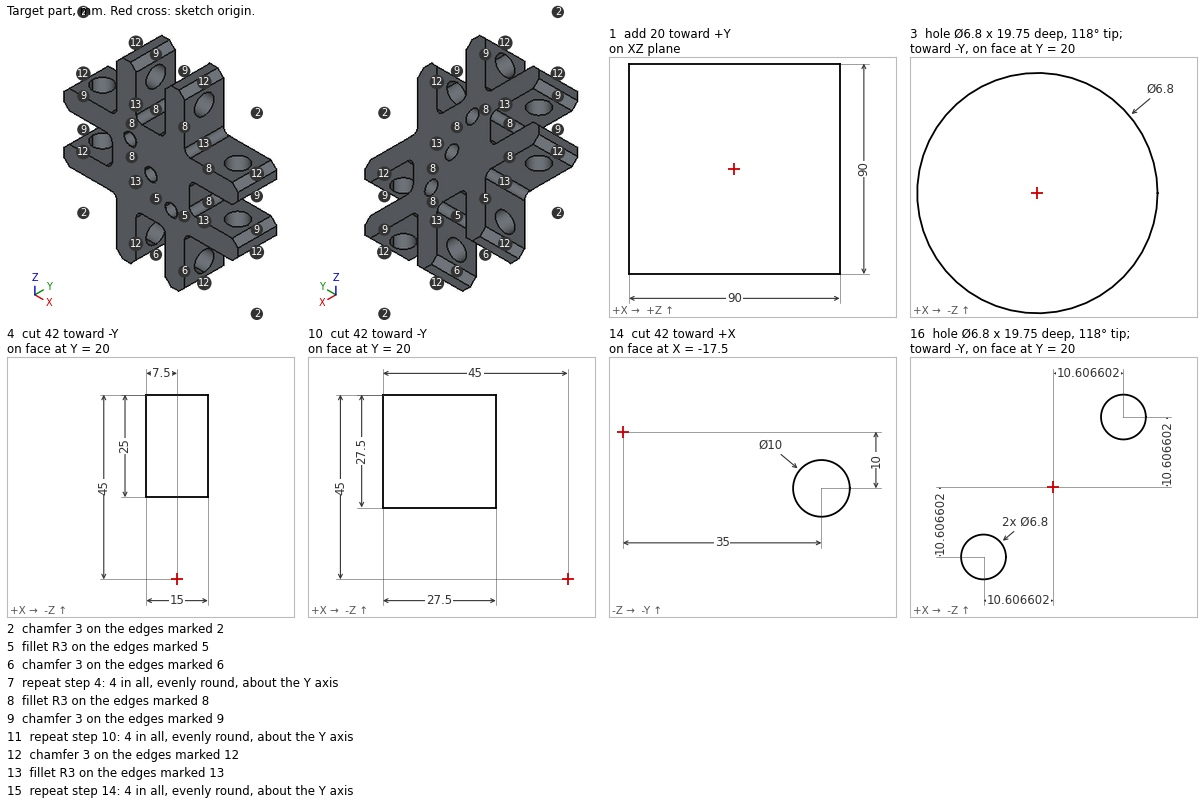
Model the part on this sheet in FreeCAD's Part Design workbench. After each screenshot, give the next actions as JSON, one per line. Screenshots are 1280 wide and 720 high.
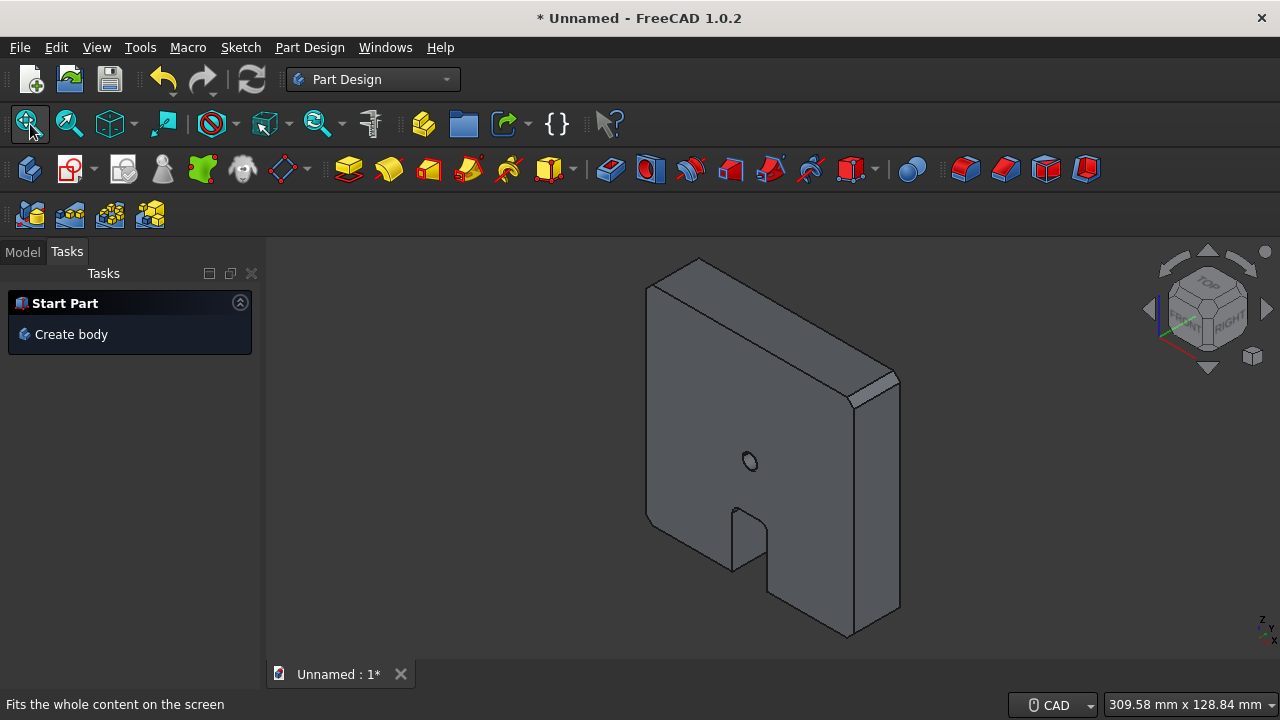
{"action": "key", "text": "1"}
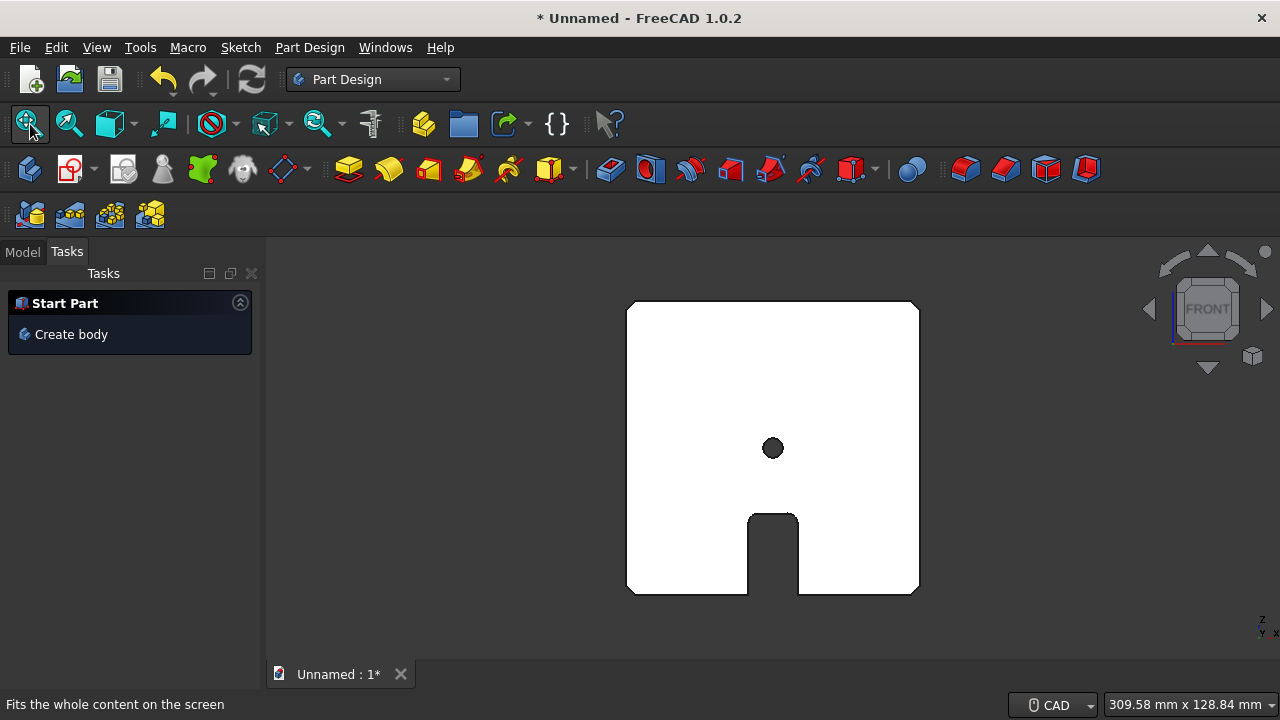
{"action": "key", "text": "3"}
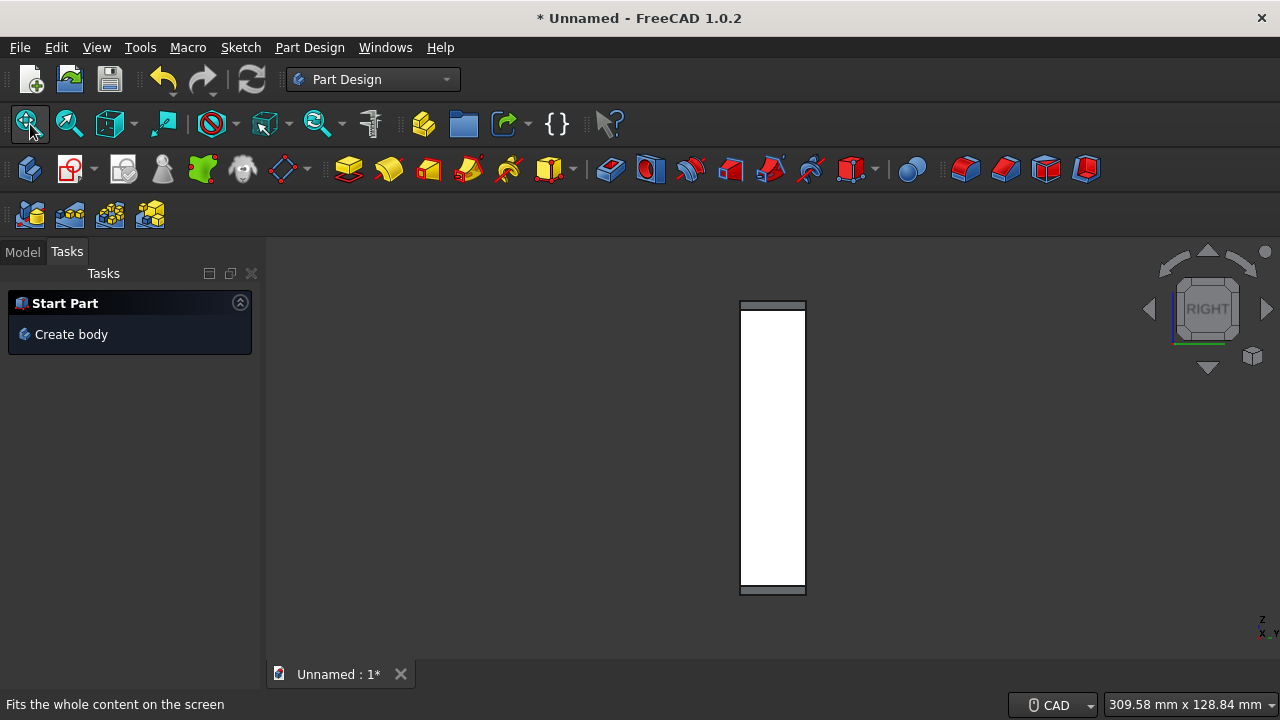
{"action": "key", "text": "5"}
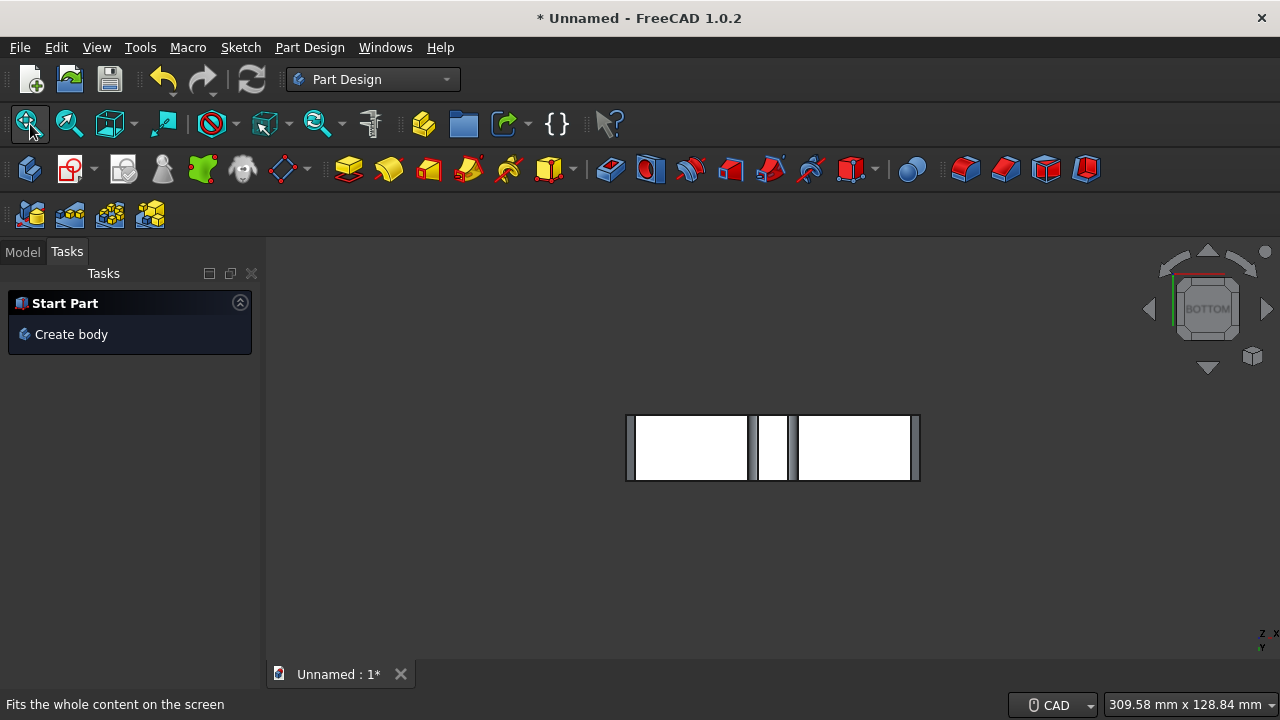
{"action": "left_click", "coordinate": [30, 124]}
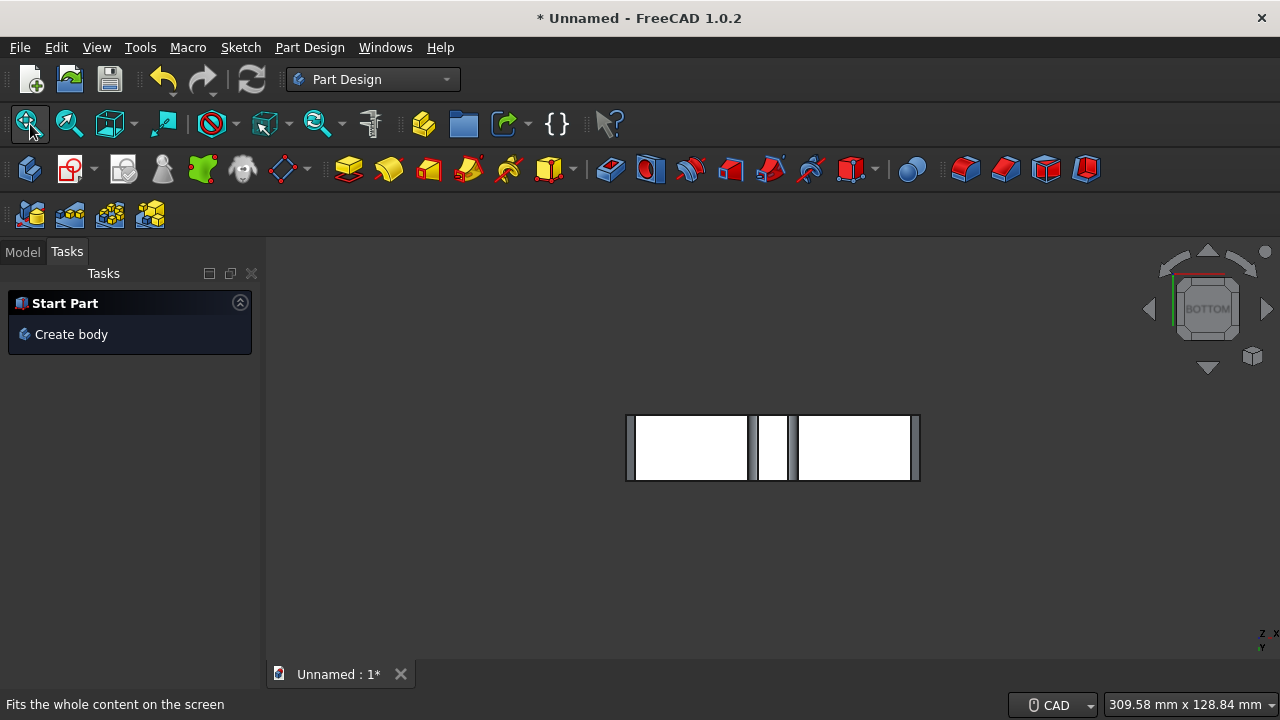
{"action": "left_click", "coordinate": [798, 447]}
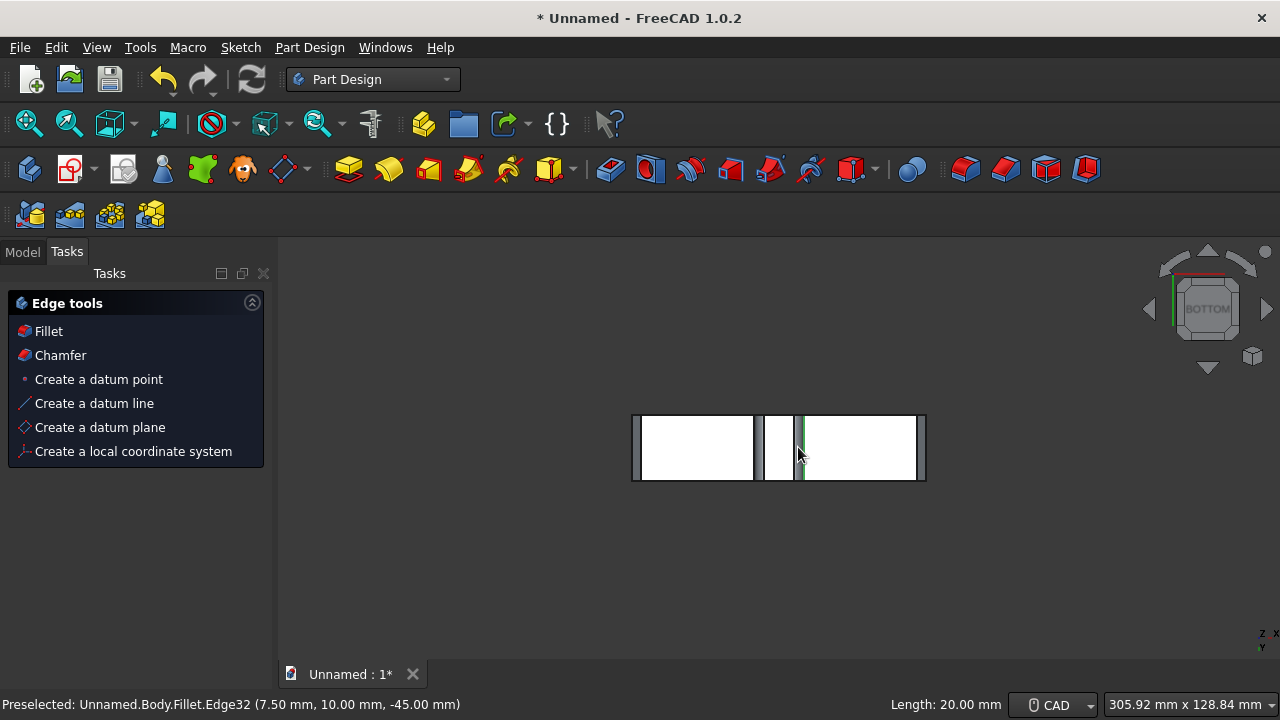
{"action": "left_click", "coordinate": [754, 447], "text": "ctrl"}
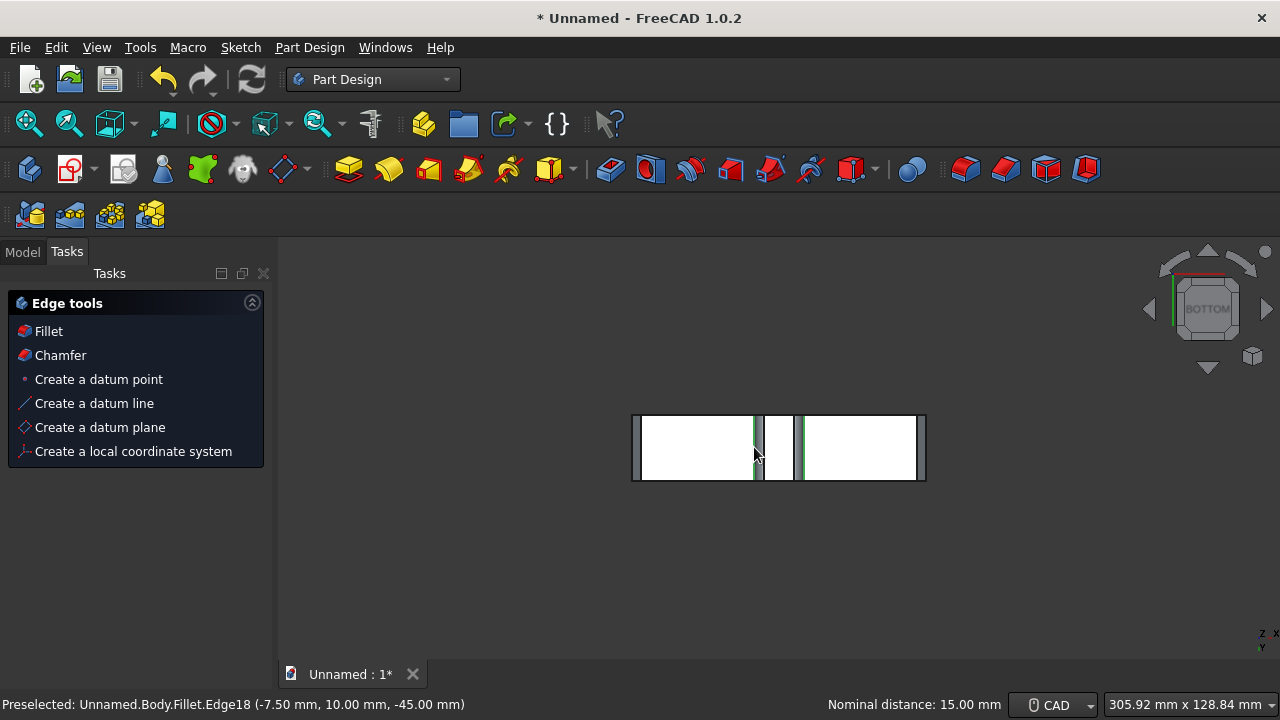
{"action": "left_click", "coordinate": [1006, 170]}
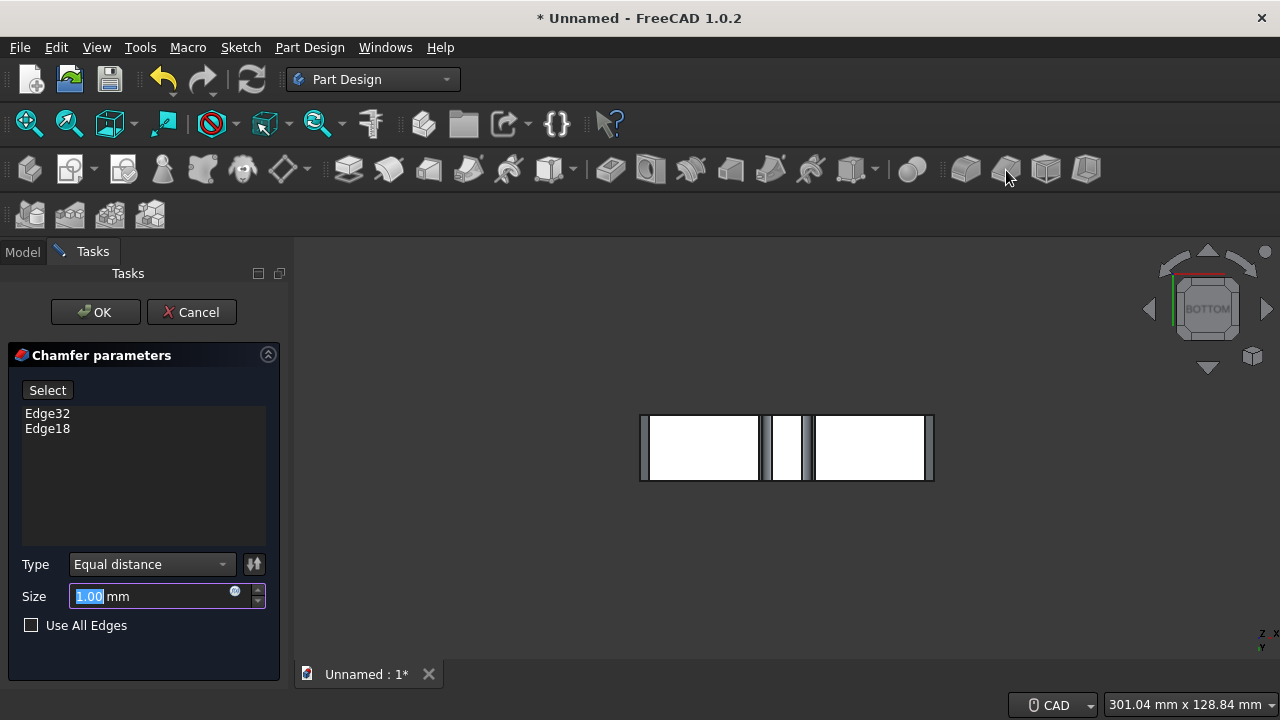
{"action": "type", "text": "3"}
{"action": "key", "text": "Tab"}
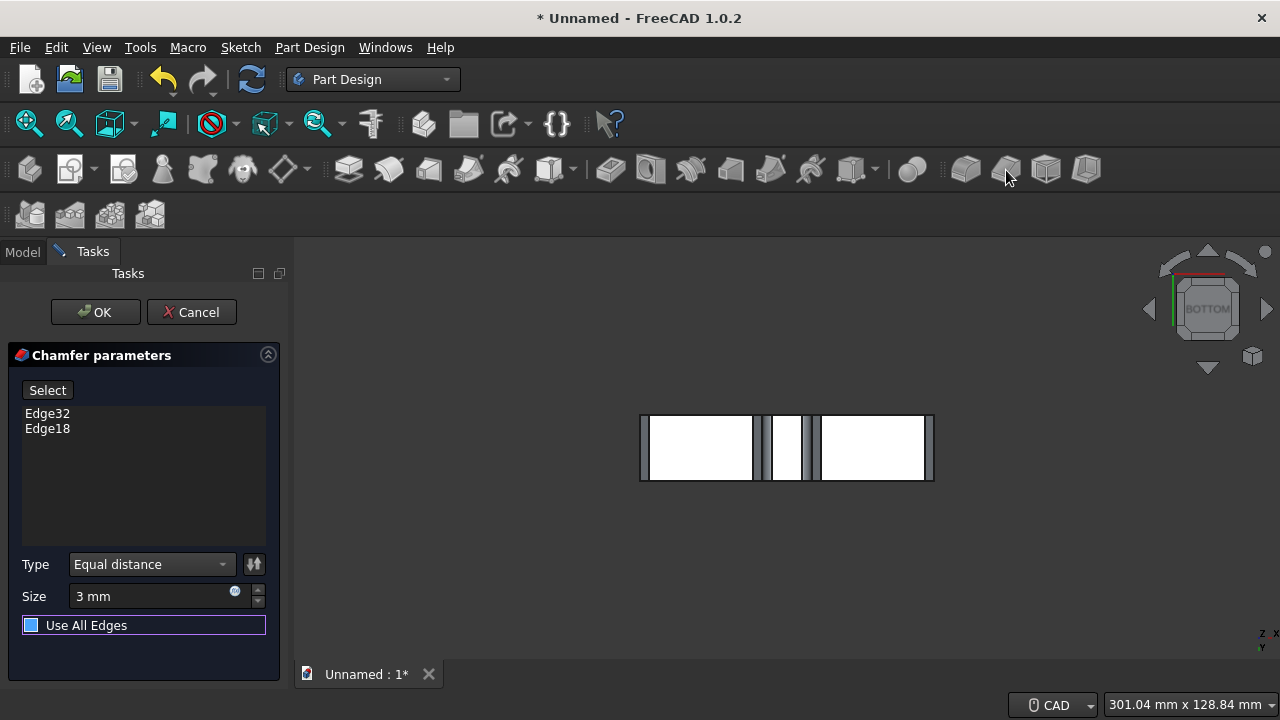
{"action": "left_click", "coordinate": [96, 312]}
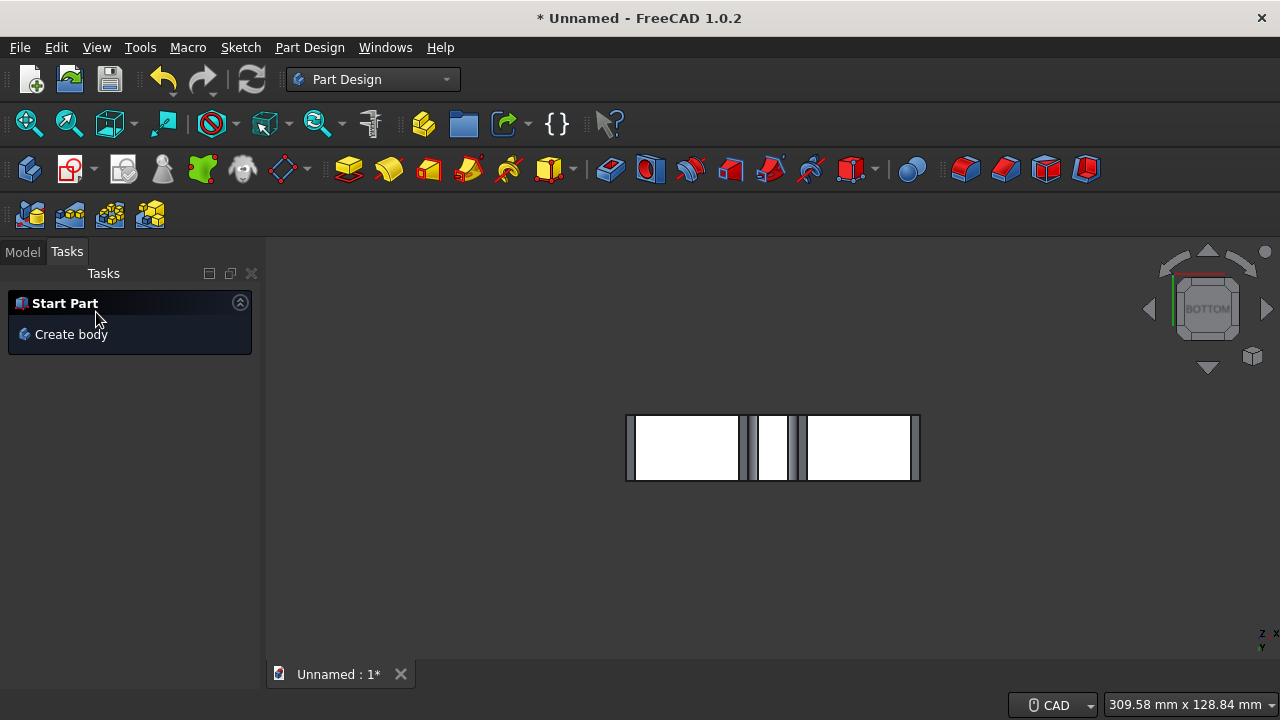
{"action": "left_click", "coordinate": [30, 124]}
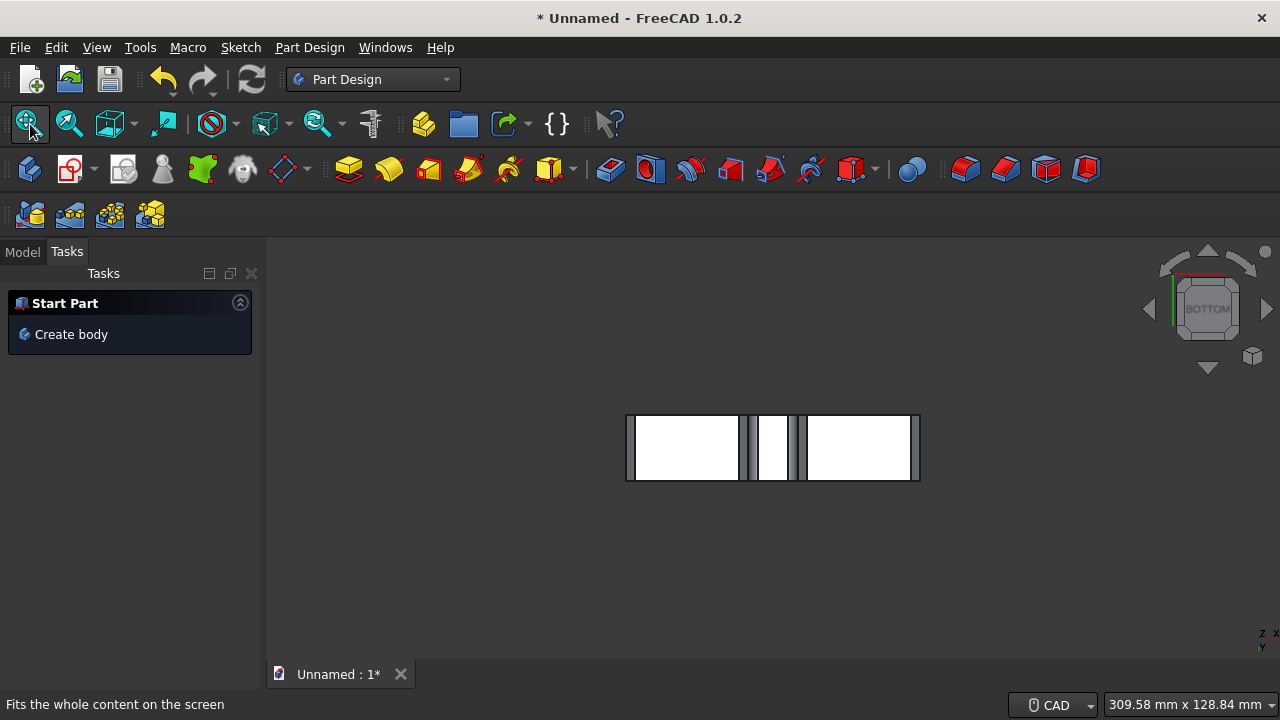
{"action": "left_click", "coordinate": [23, 251]}